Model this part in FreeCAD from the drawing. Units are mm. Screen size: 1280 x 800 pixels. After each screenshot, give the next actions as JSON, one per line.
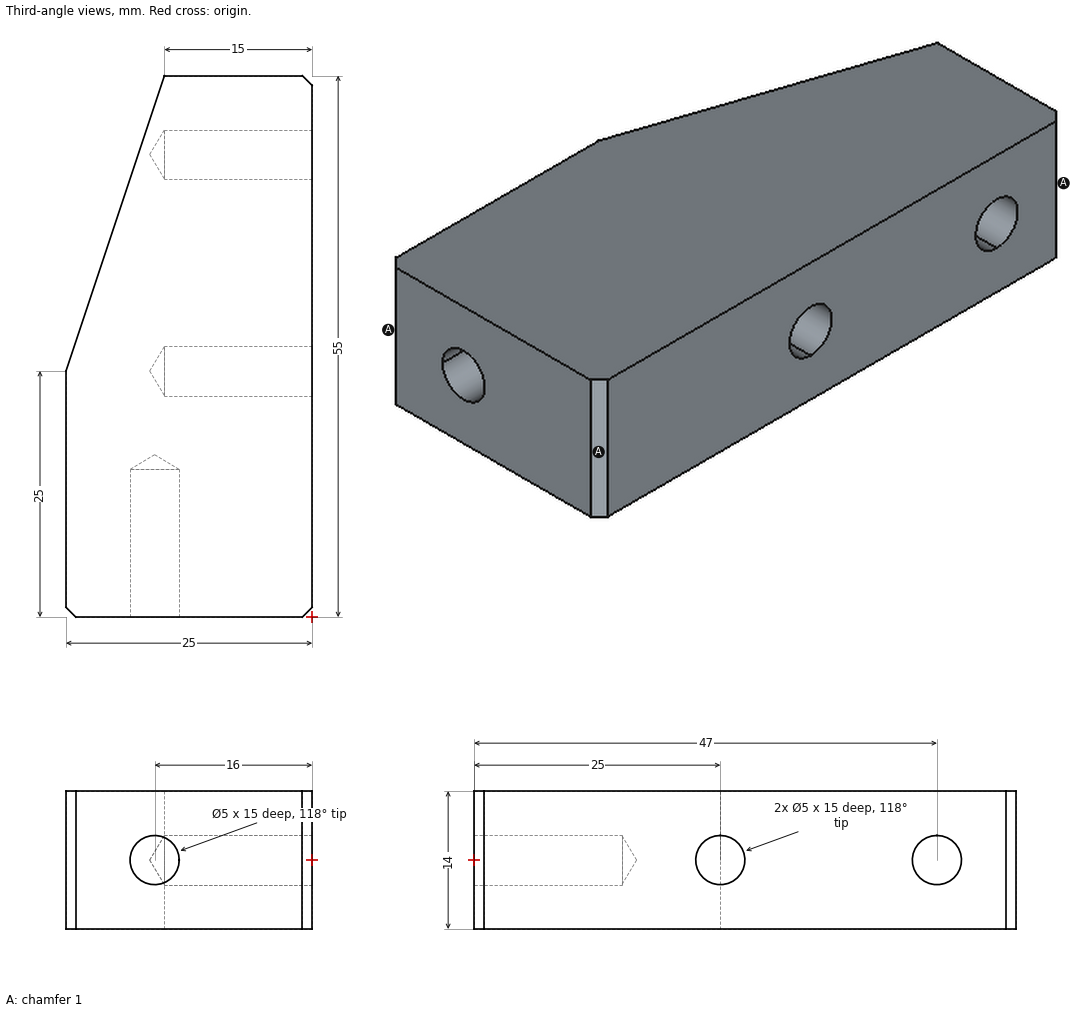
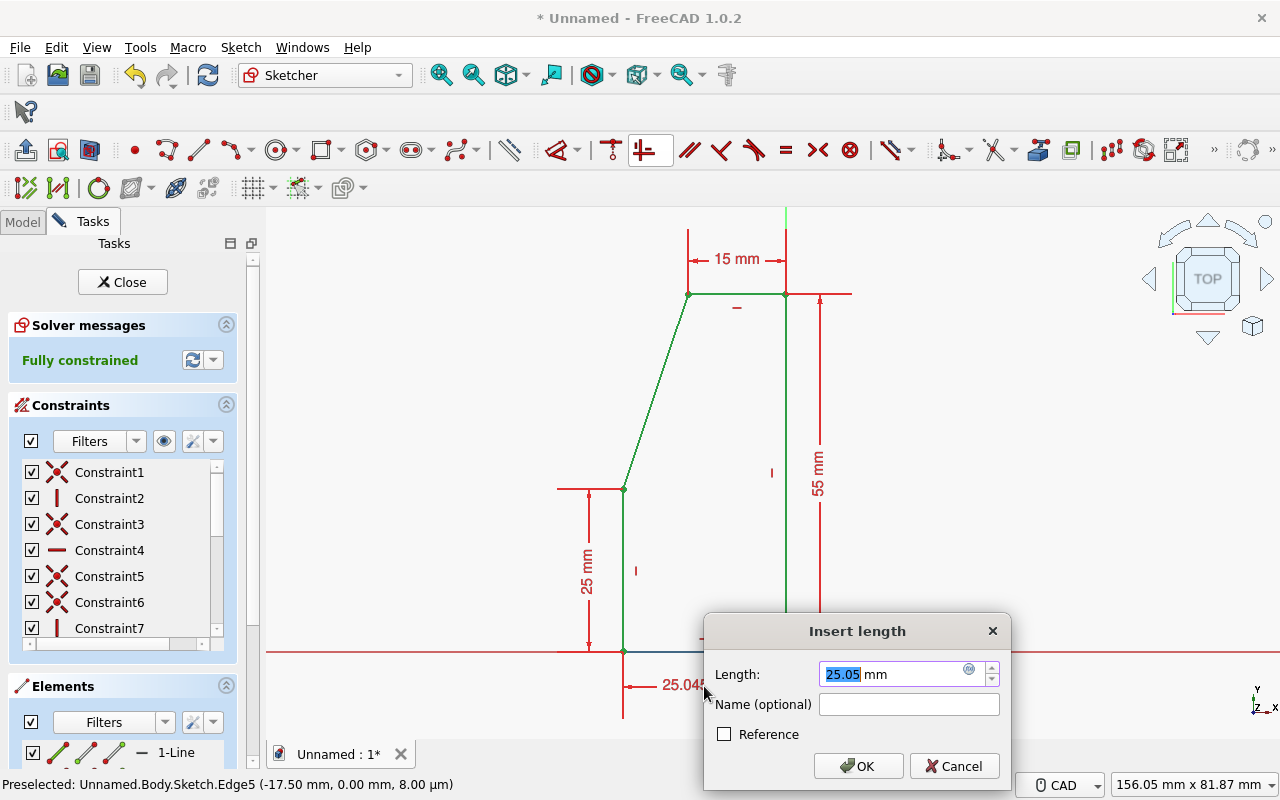
{"action": "type", "text": "25"}
{"action": "key", "text": "Return"}
{"action": "key", "text": "Escape"}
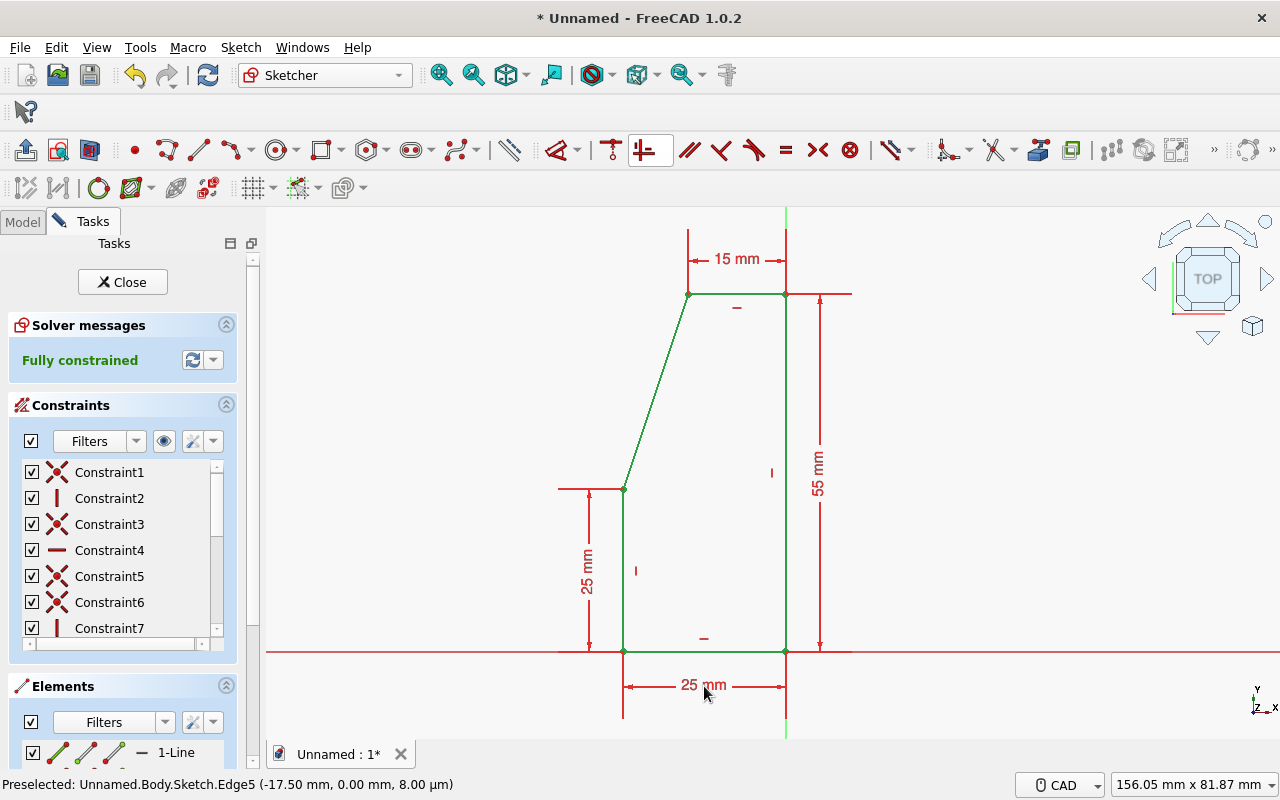
{"action": "left_click", "coordinate": [123, 282]}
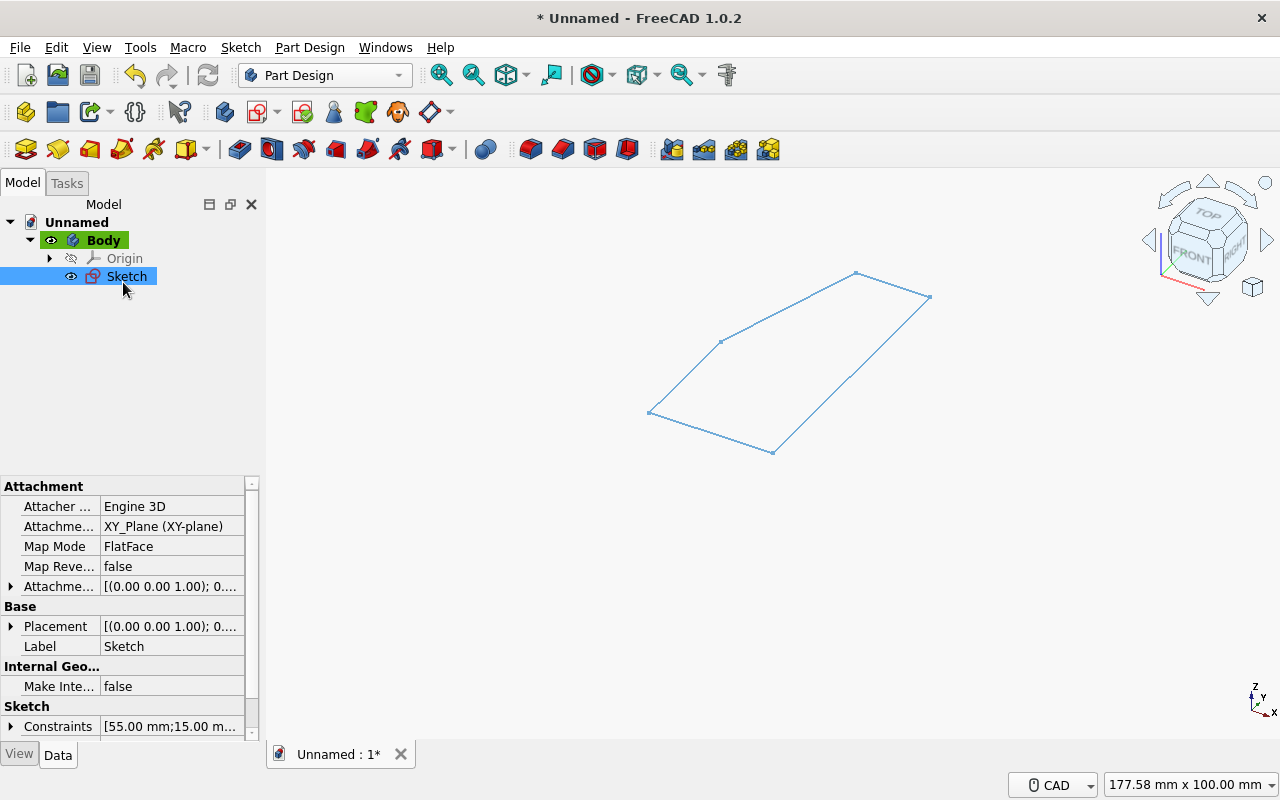
{"action": "left_click", "coordinate": [26, 150]}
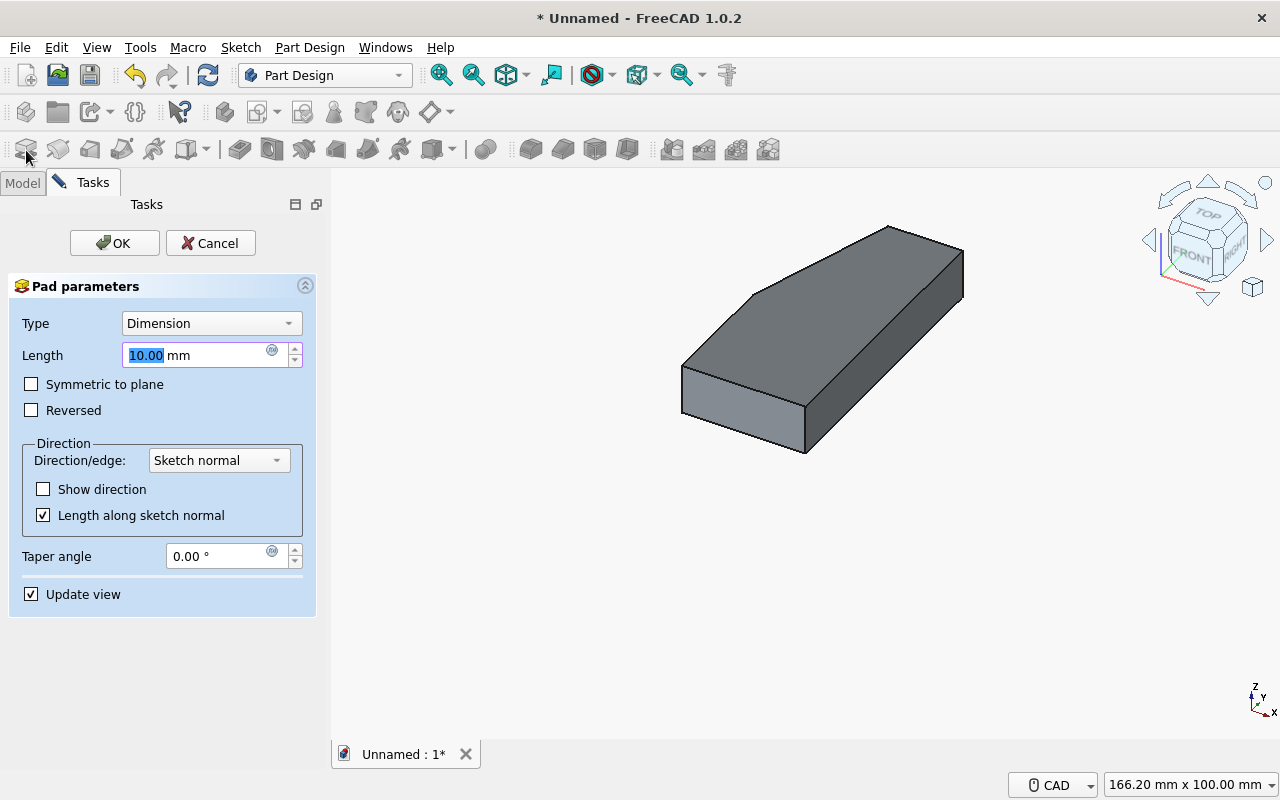
{"action": "type", "text": "14"}
{"action": "key", "text": "Tab"}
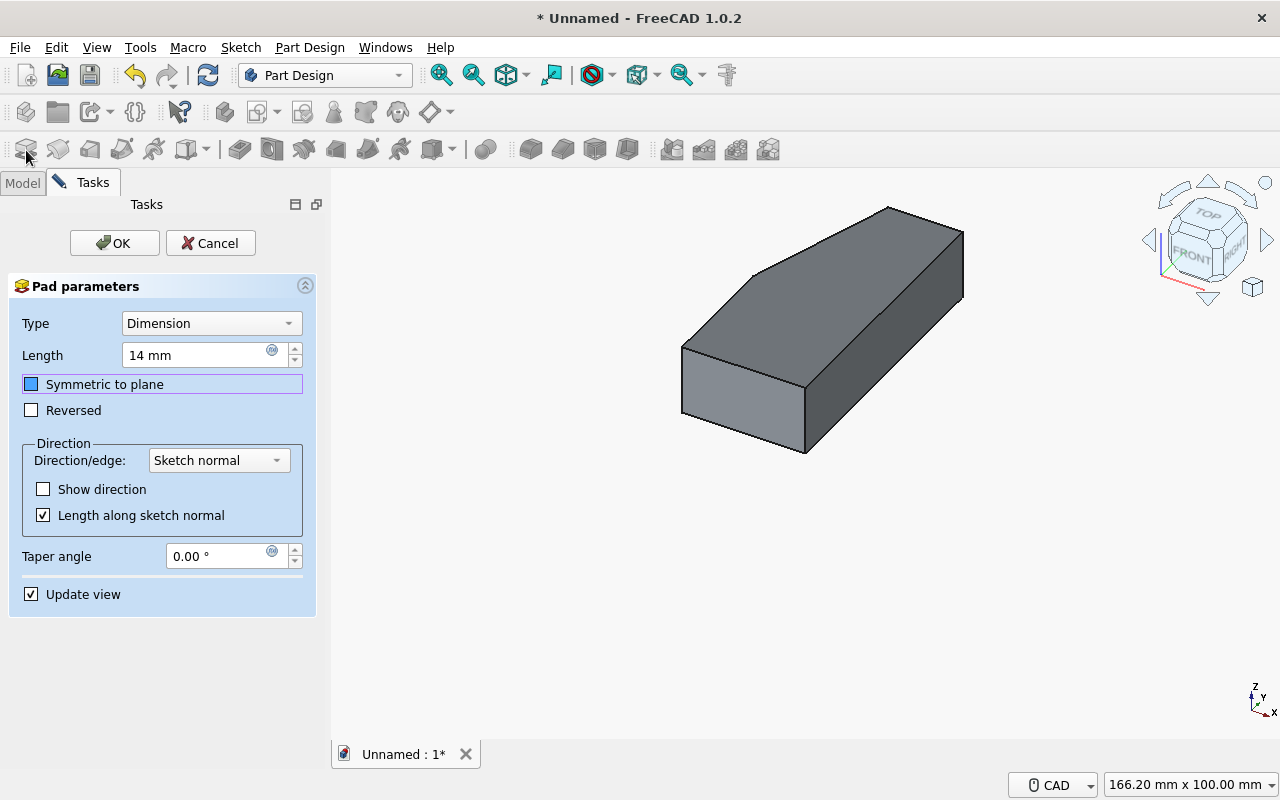
{"action": "left_click", "coordinate": [30, 384]}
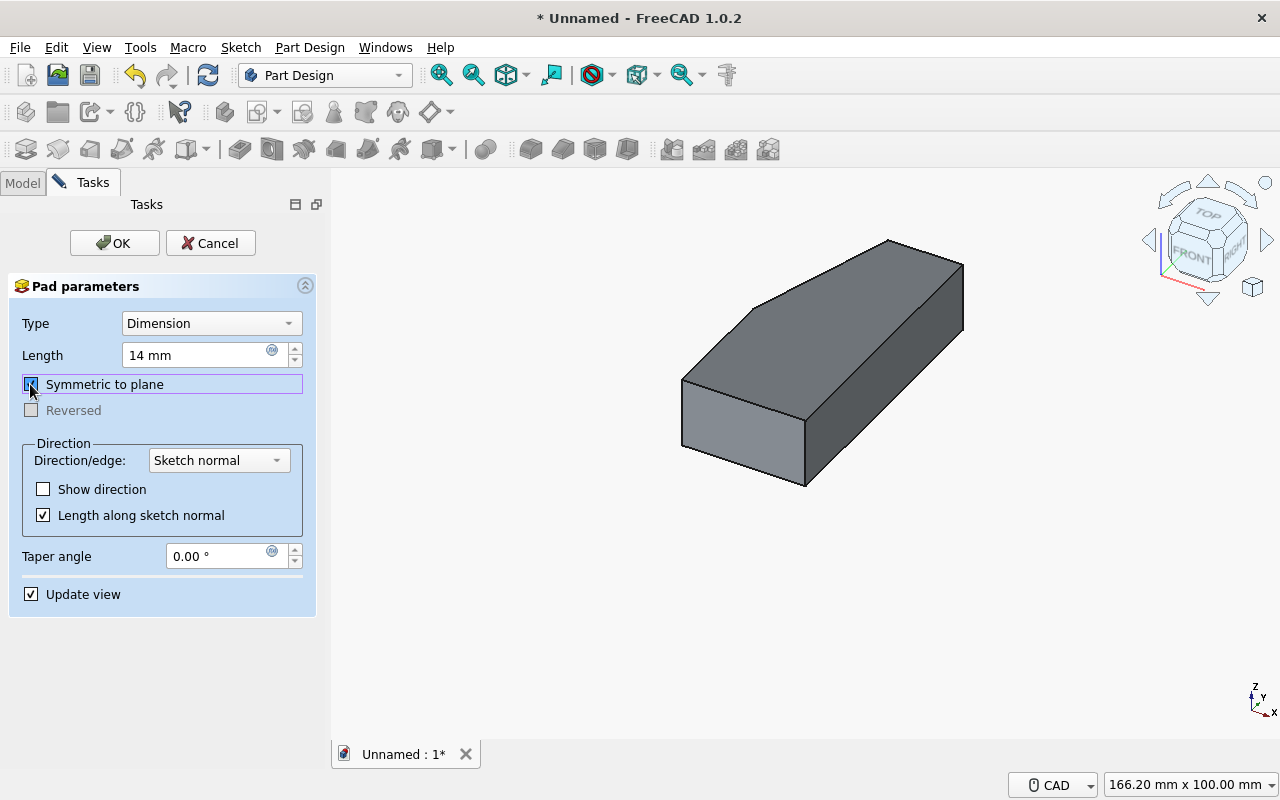
{"action": "left_click", "coordinate": [115, 243]}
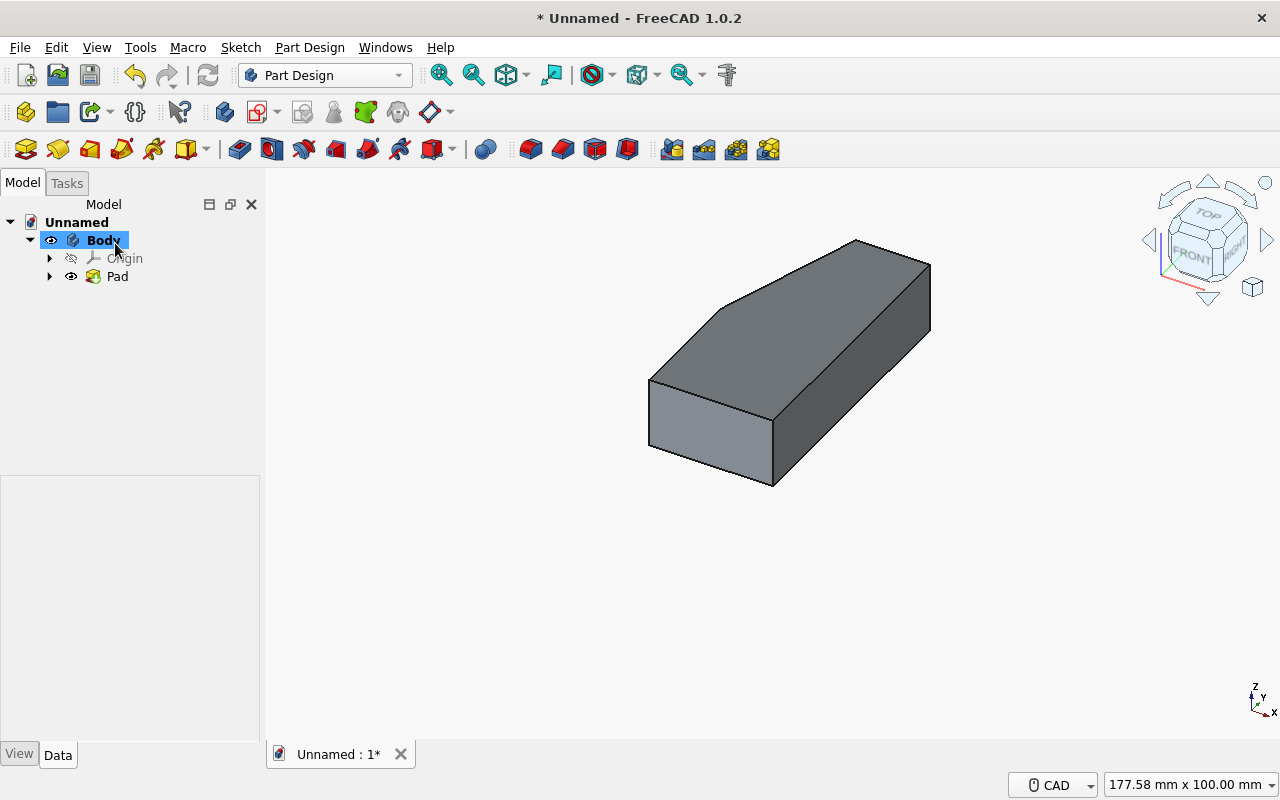
{"action": "left_click", "coordinate": [896, 330]}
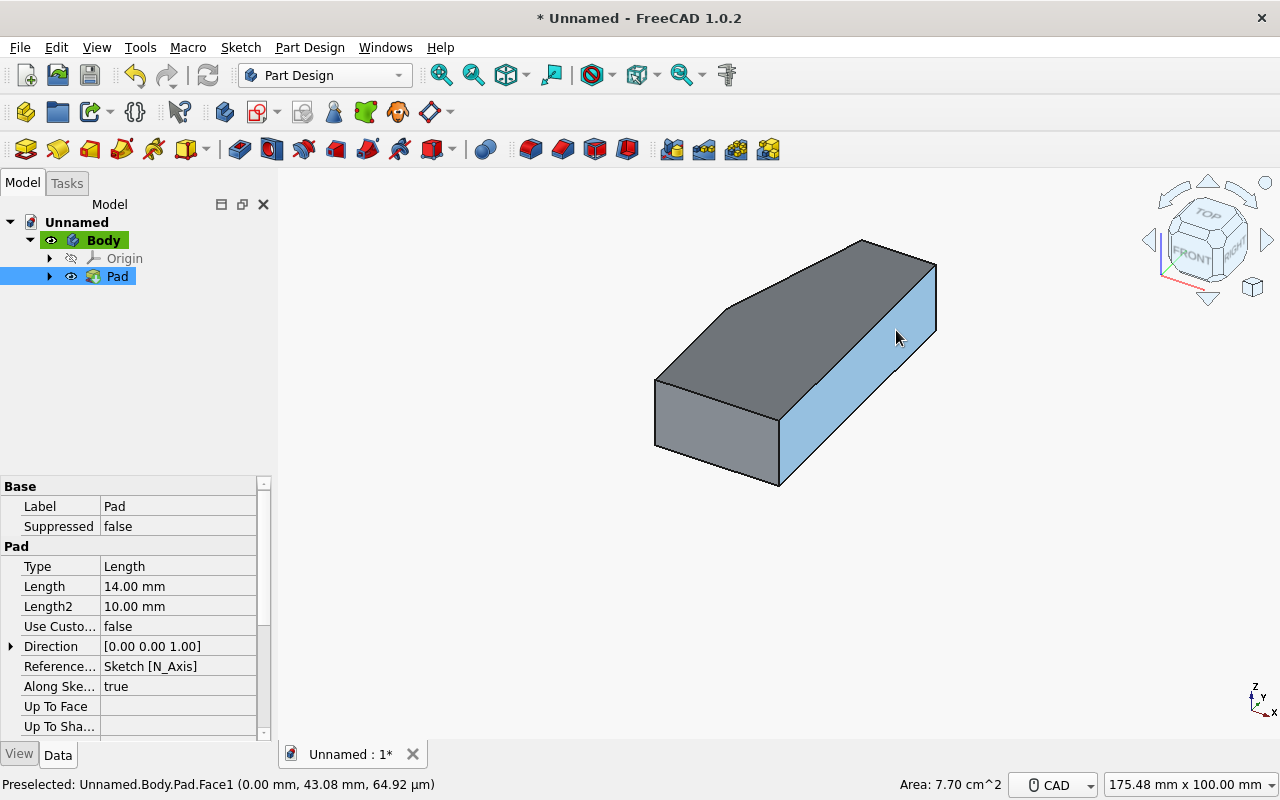
{"action": "left_click", "coordinate": [258, 112]}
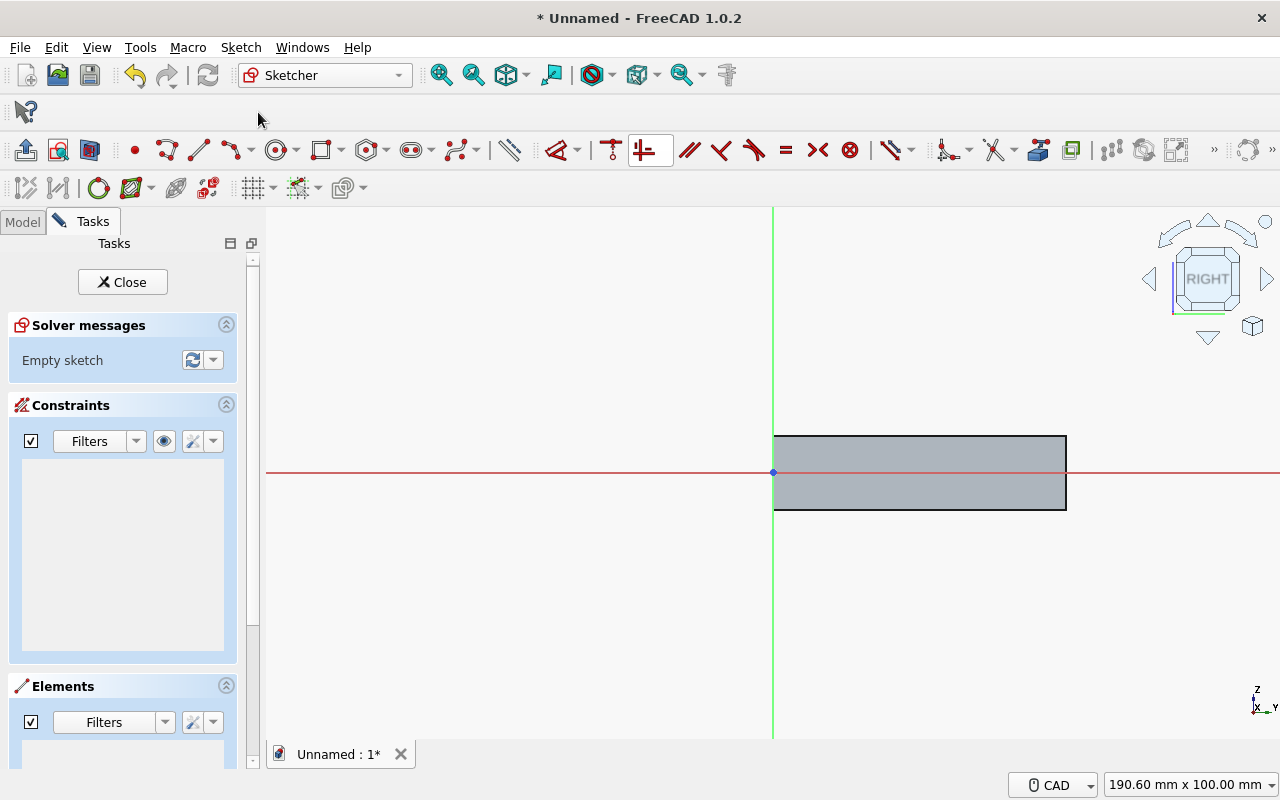
{"action": "scroll", "coordinate": [1068, 473], "scroll_direction": "up", "scroll_amount": 4}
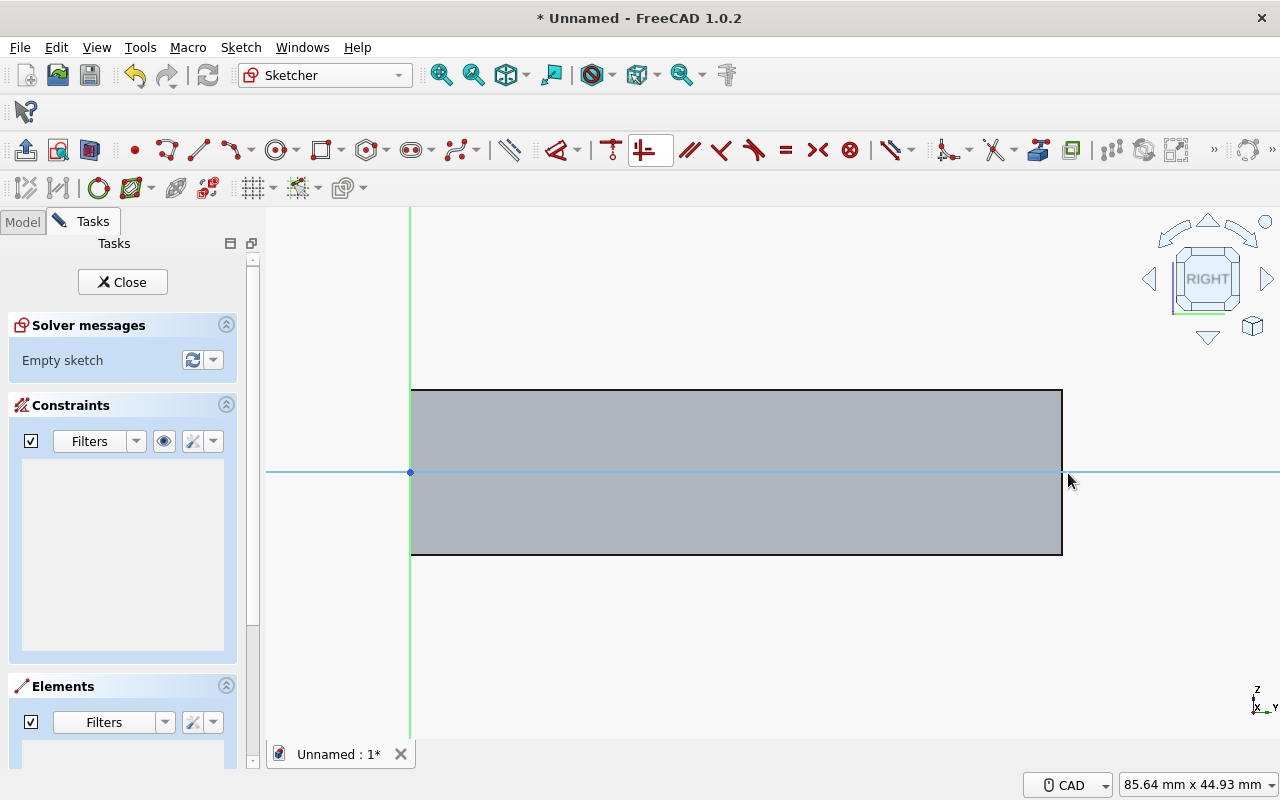
{"action": "left_click", "coordinate": [276, 150]}